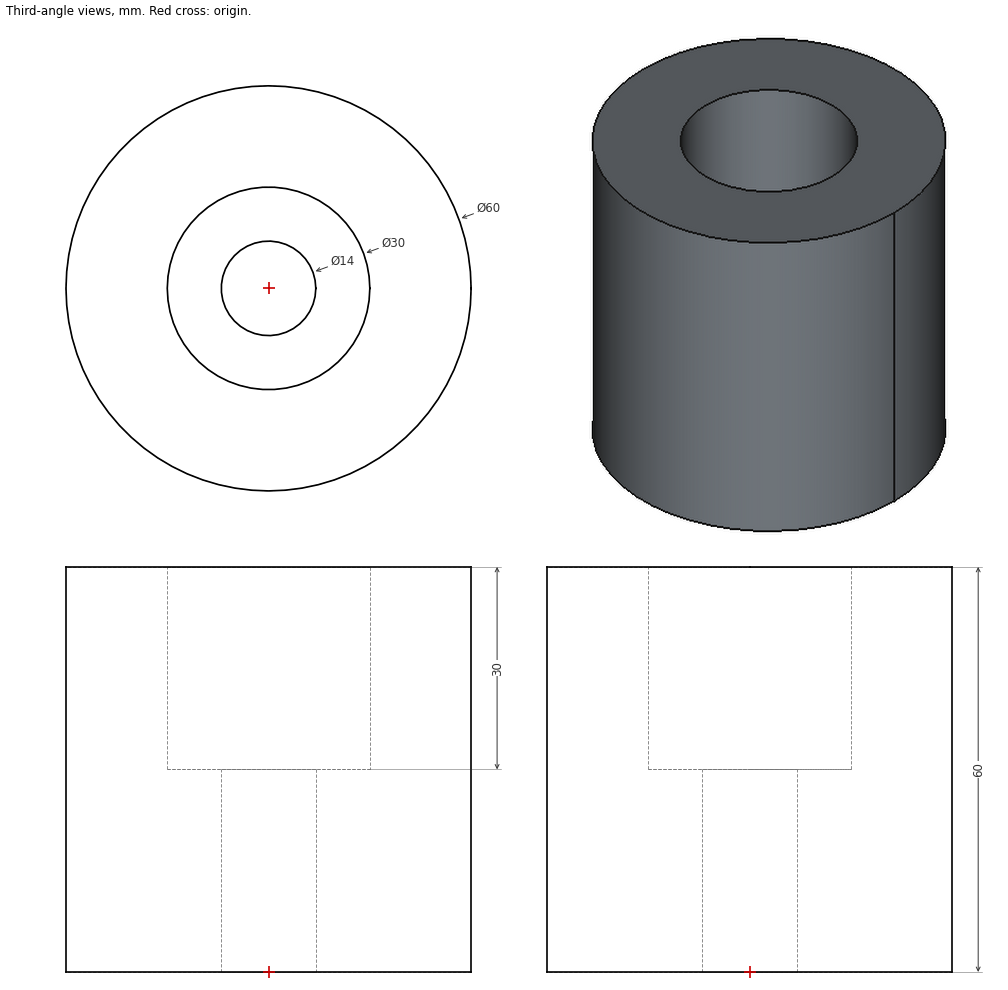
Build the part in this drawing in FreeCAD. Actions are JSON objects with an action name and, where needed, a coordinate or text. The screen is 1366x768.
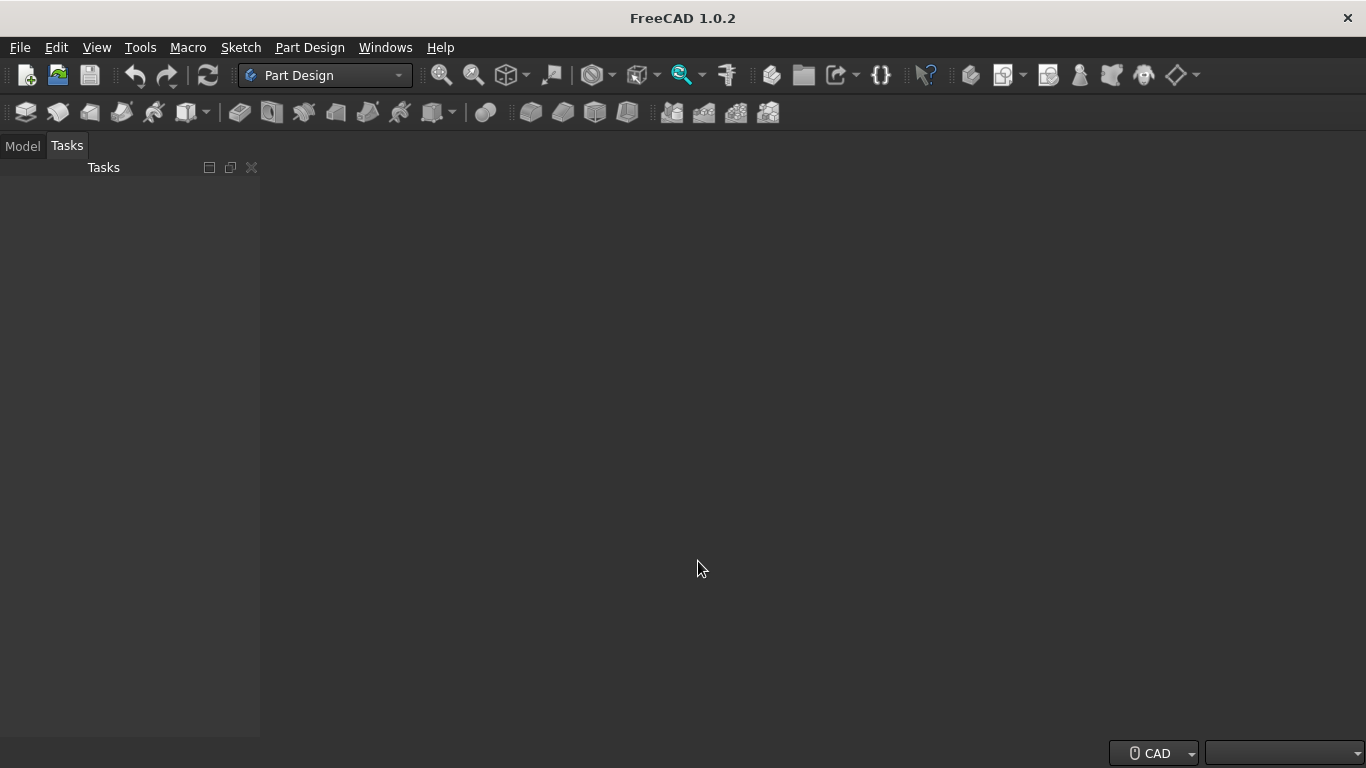
{"action": "key", "text": "ctrl+n"}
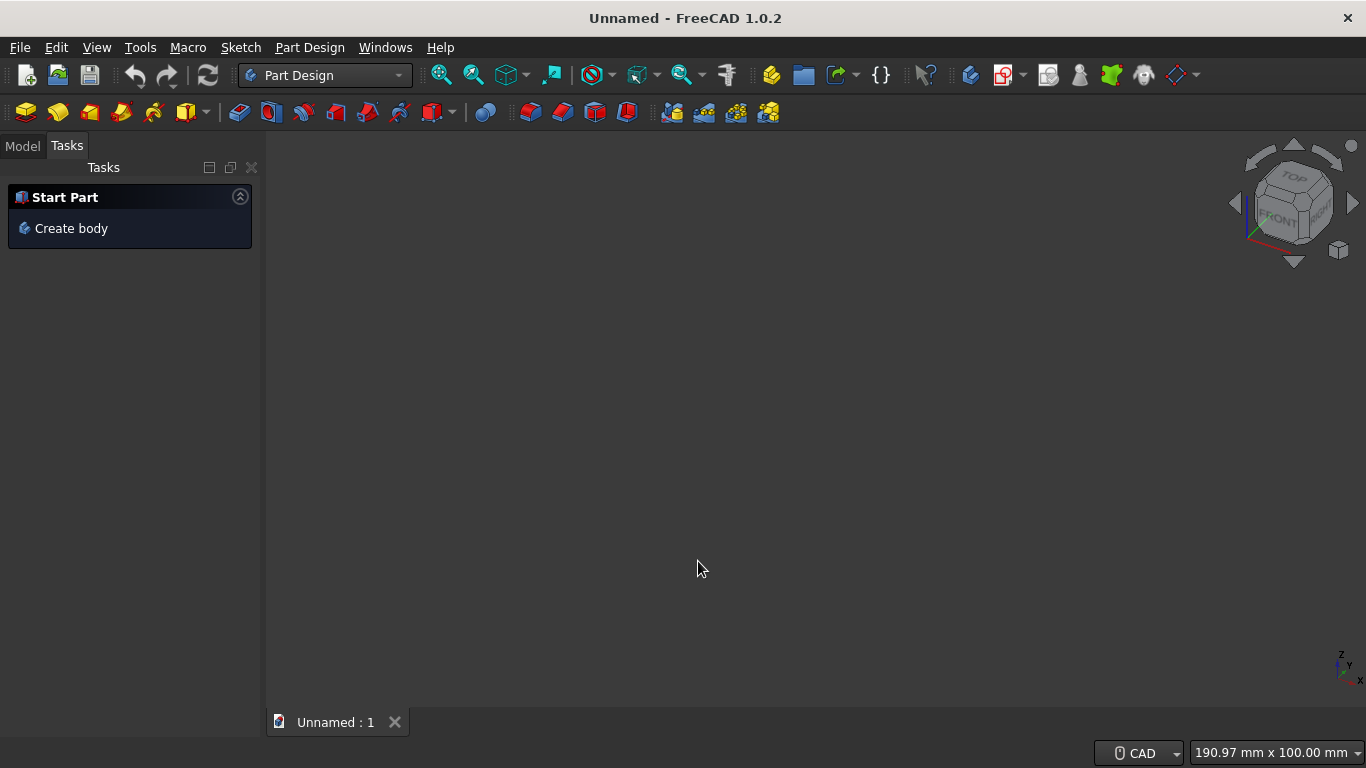
{"action": "left_click", "coordinate": [1004, 76]}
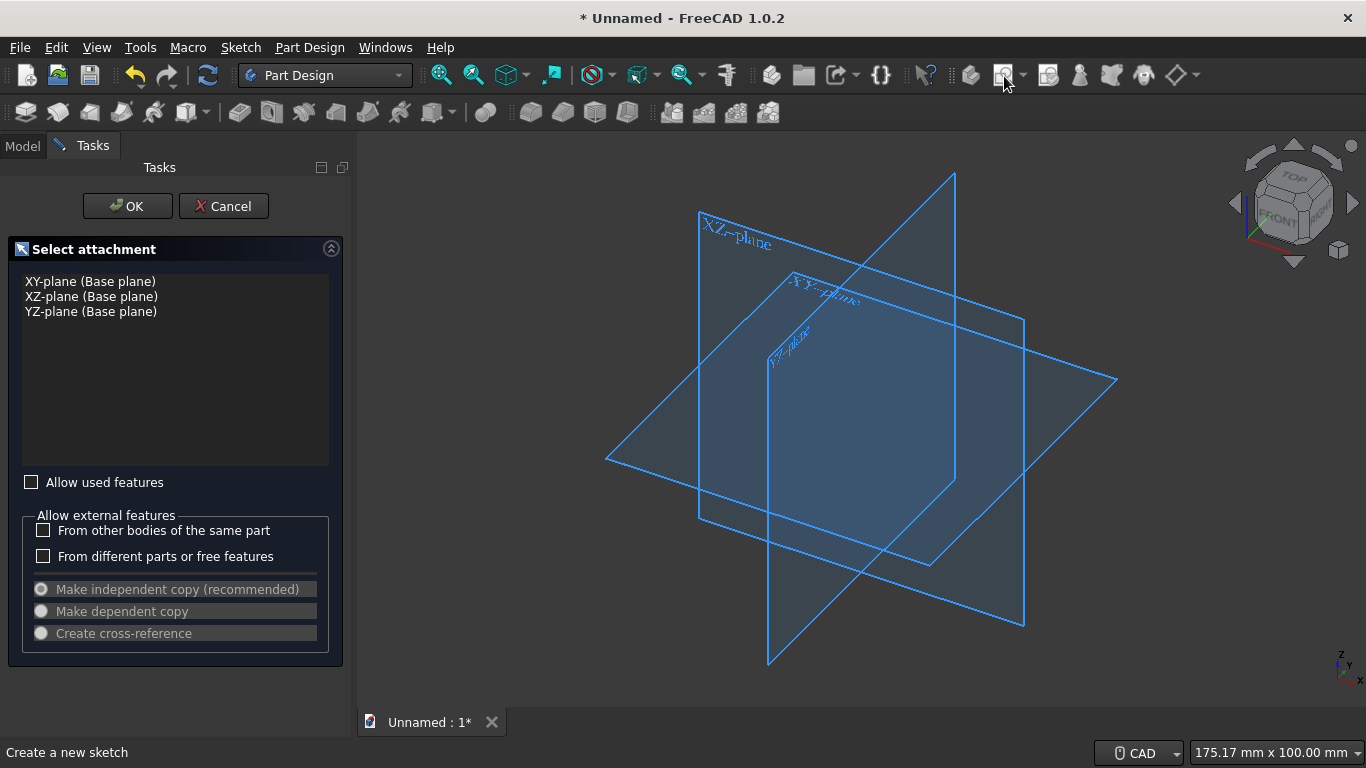
{"action": "left_click", "coordinate": [82, 282]}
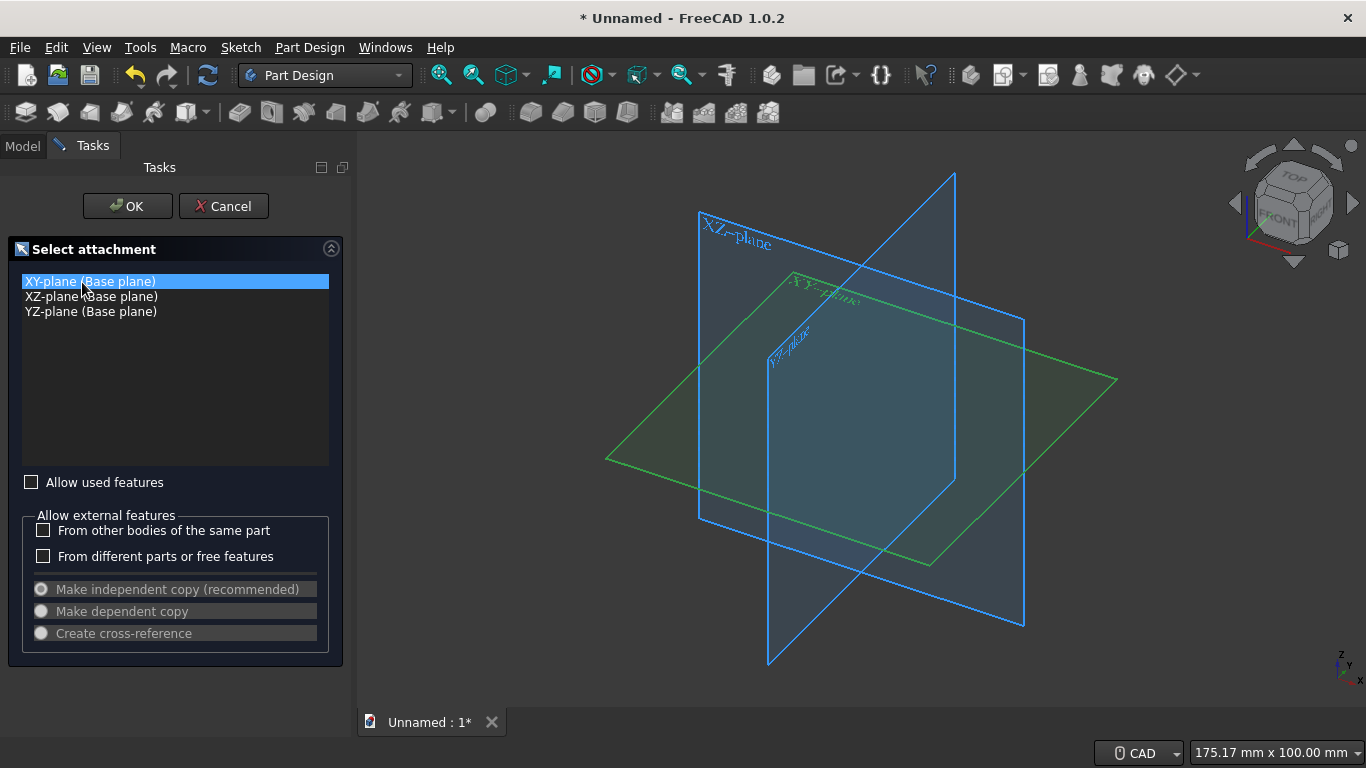
{"action": "left_click", "coordinate": [128, 206]}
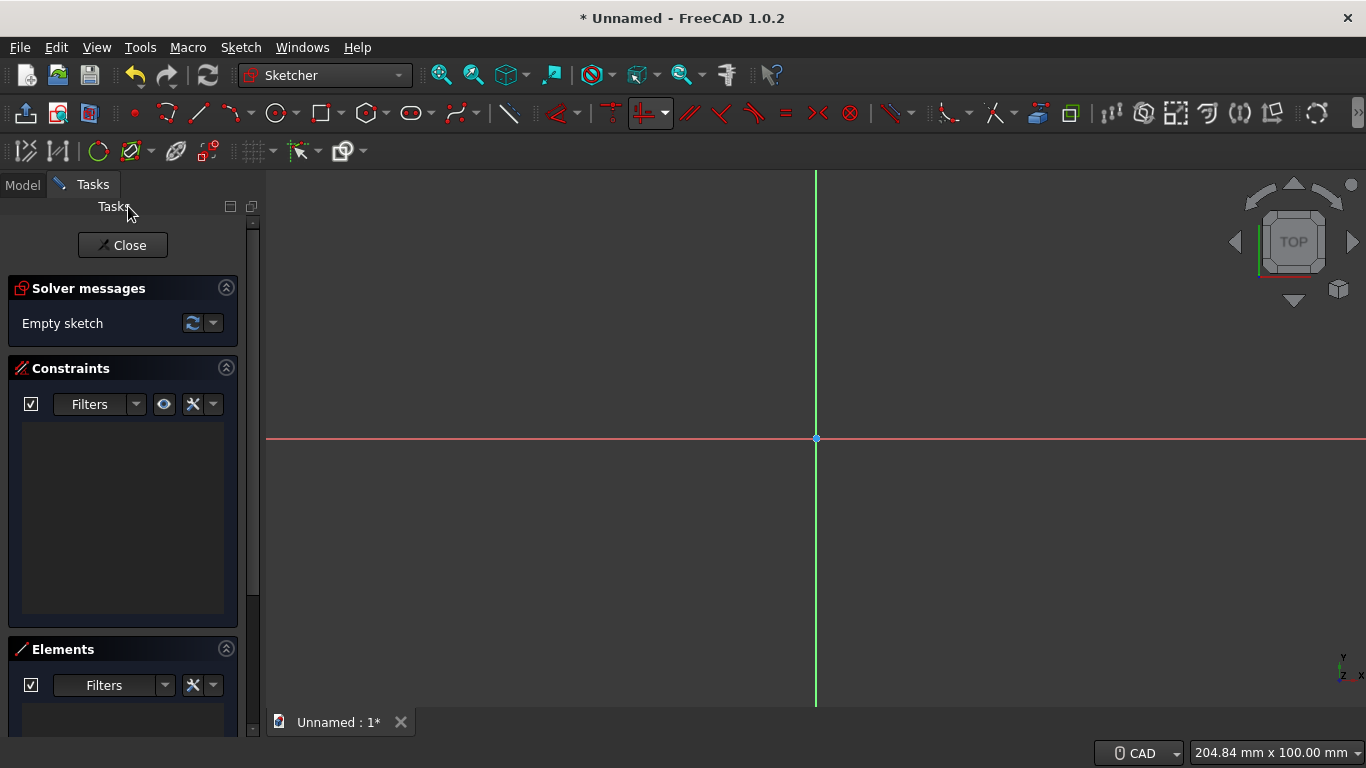
{"action": "left_click", "coordinate": [276, 114]}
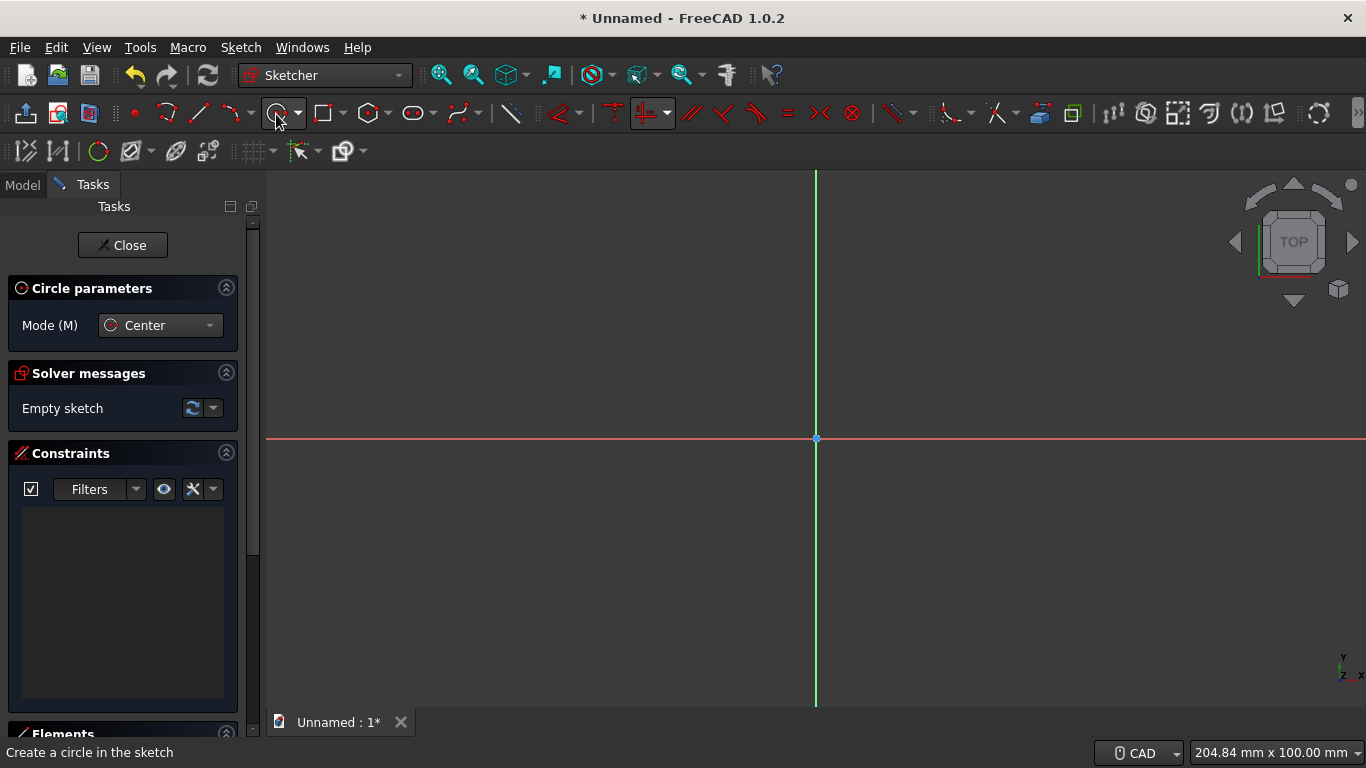
{"action": "left_click", "coordinate": [816, 438]}
{"action": "mouse_move", "coordinate": [930, 325]}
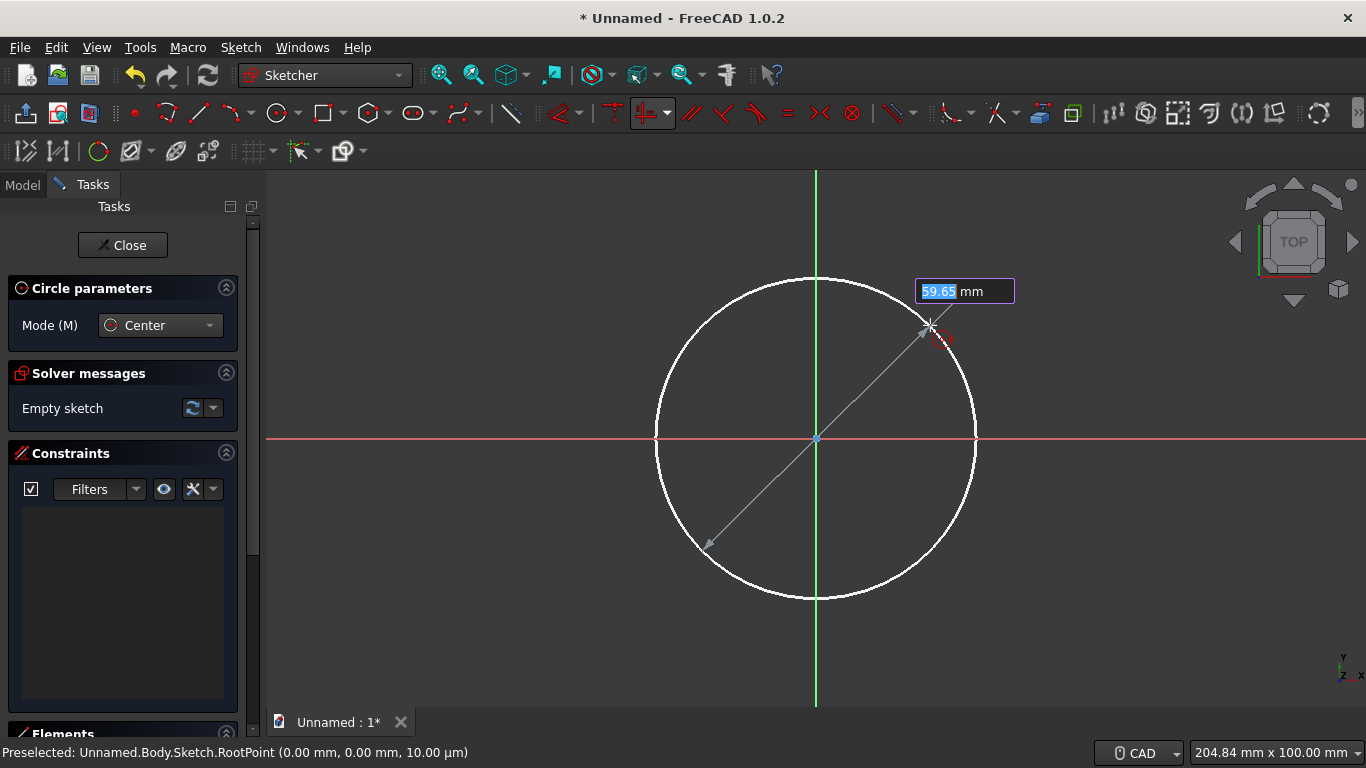
{"action": "type", "text": "60"}
{"action": "key", "text": "Return"}
{"action": "key", "text": "Escape"}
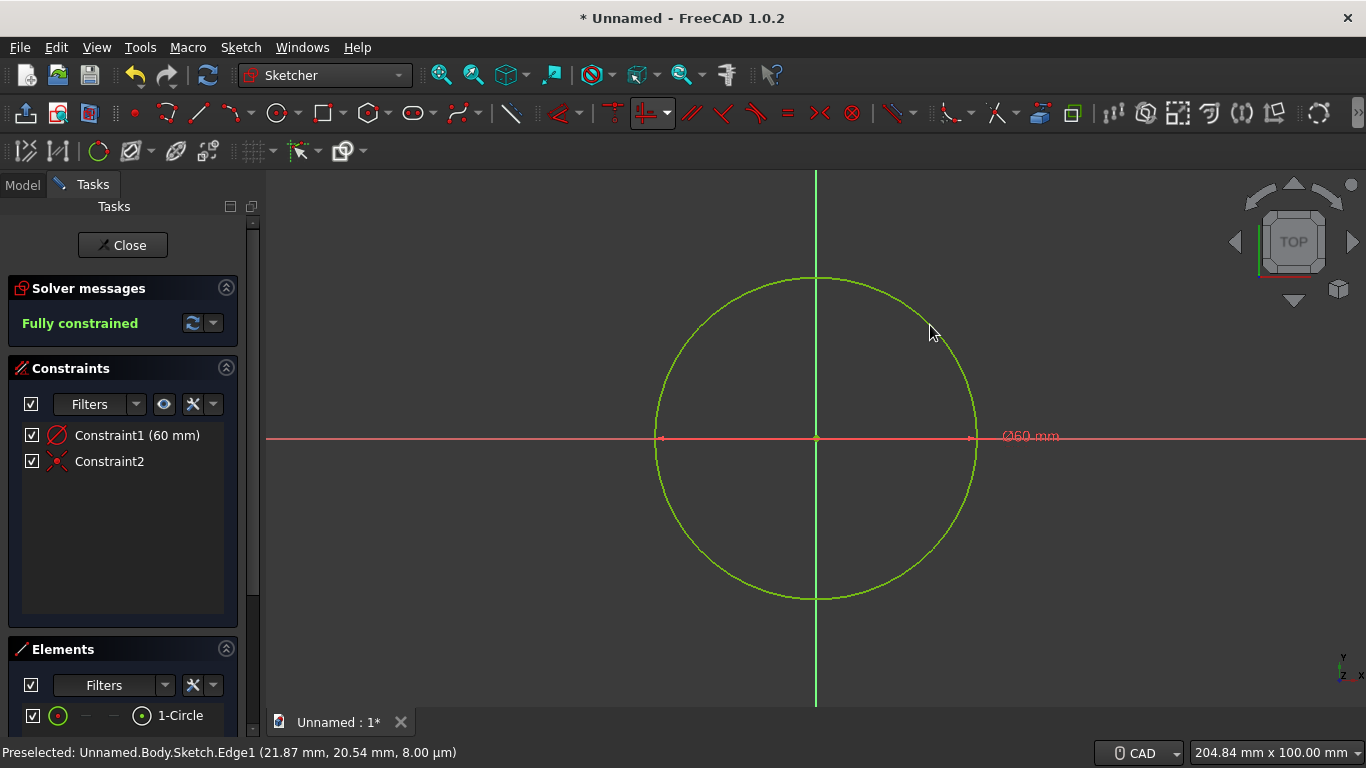
{"action": "left_click", "coordinate": [123, 245]}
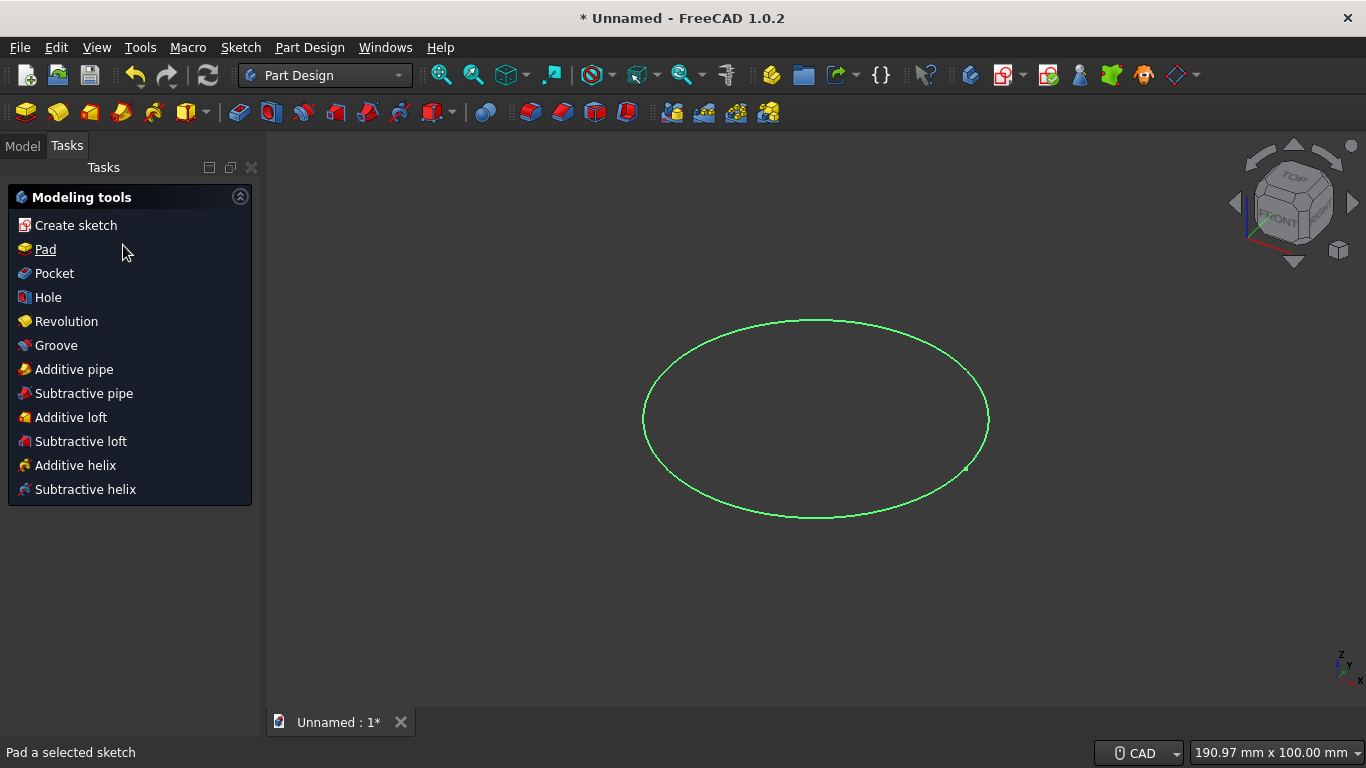
{"action": "left_click", "coordinate": [26, 112]}